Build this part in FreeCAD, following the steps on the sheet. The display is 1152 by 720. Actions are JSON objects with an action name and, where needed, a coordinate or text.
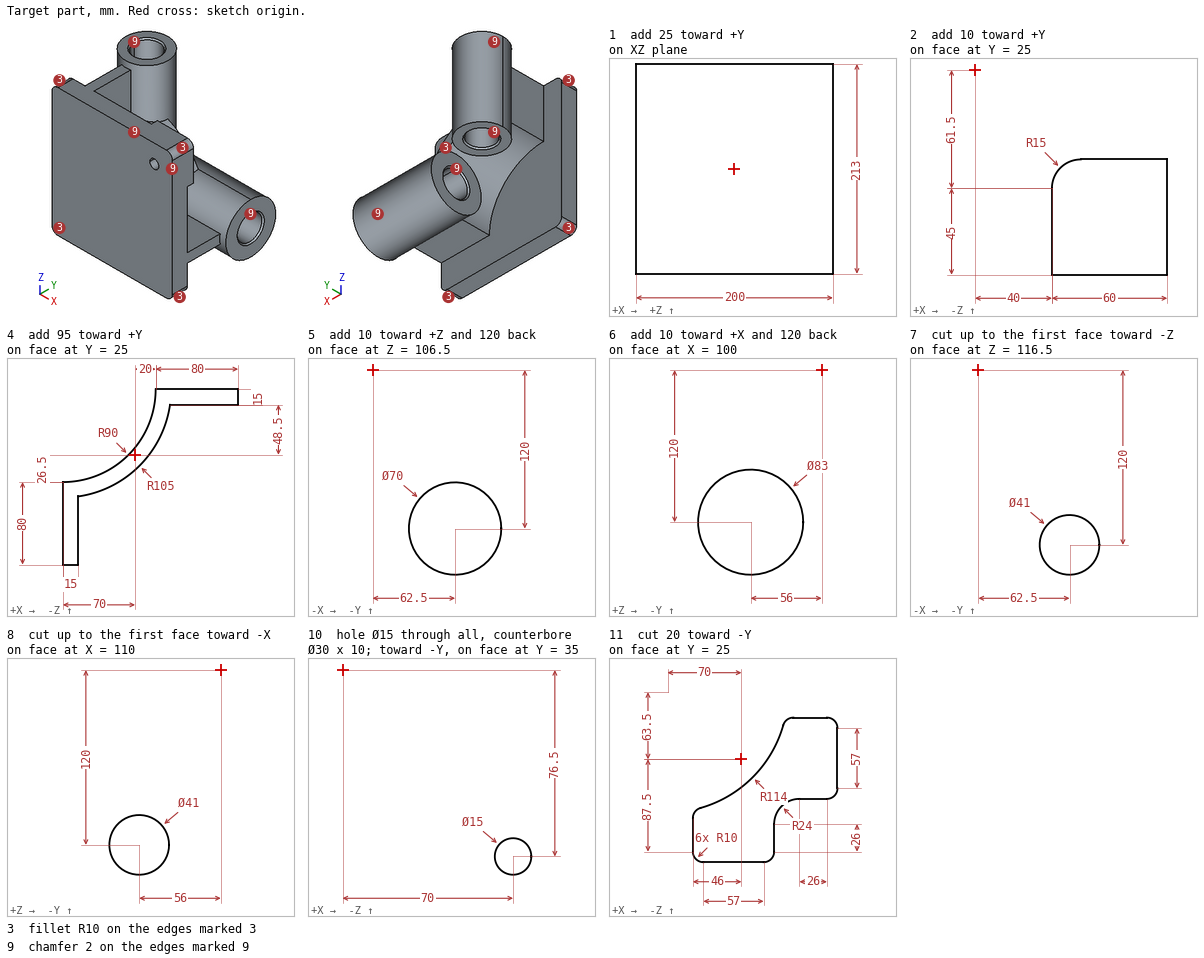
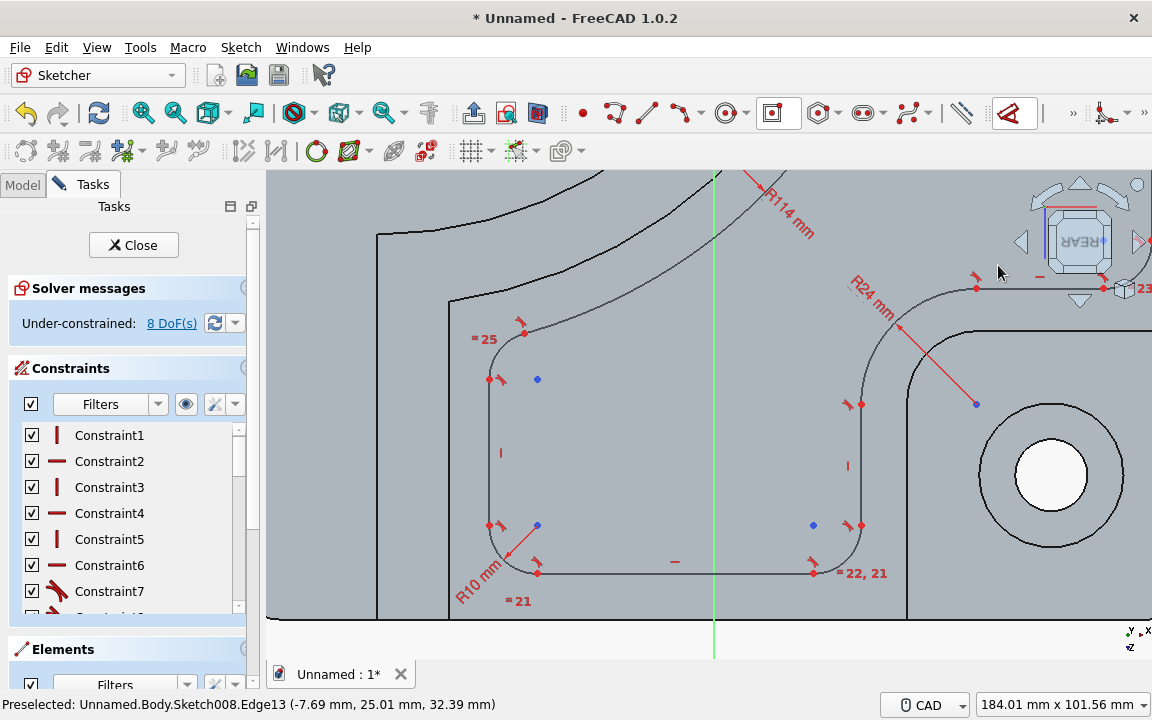
{"action": "left_click", "coordinate": [620, 574]}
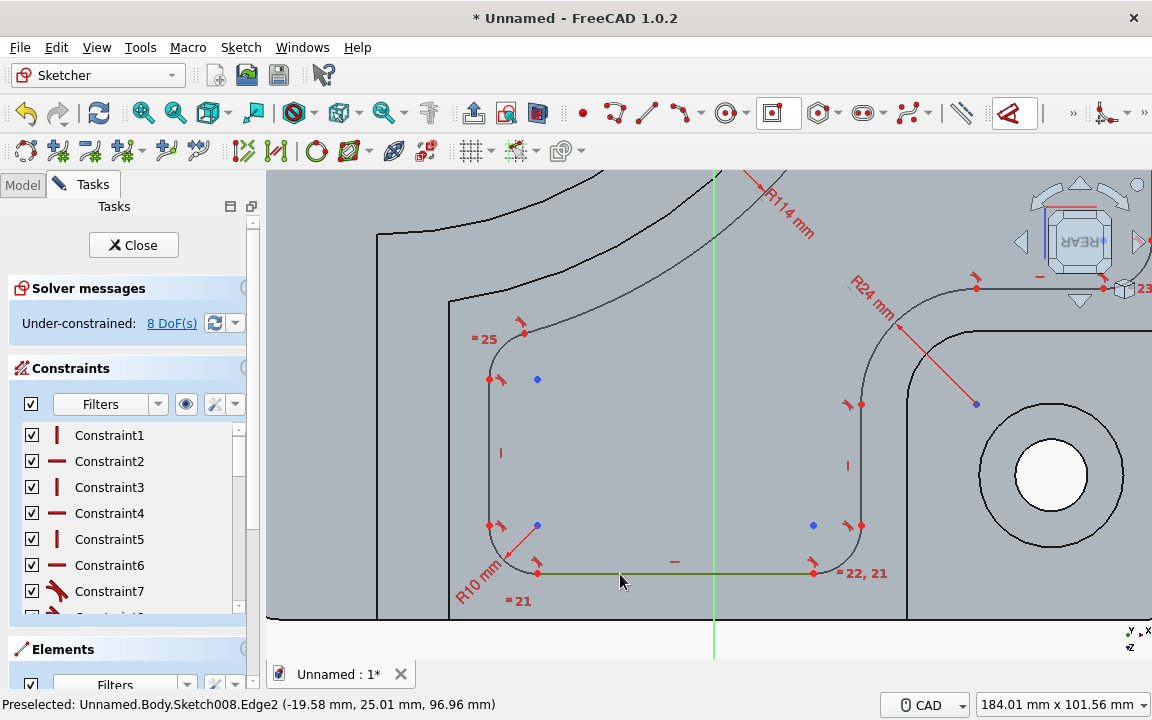
{"action": "key", "text": "l"}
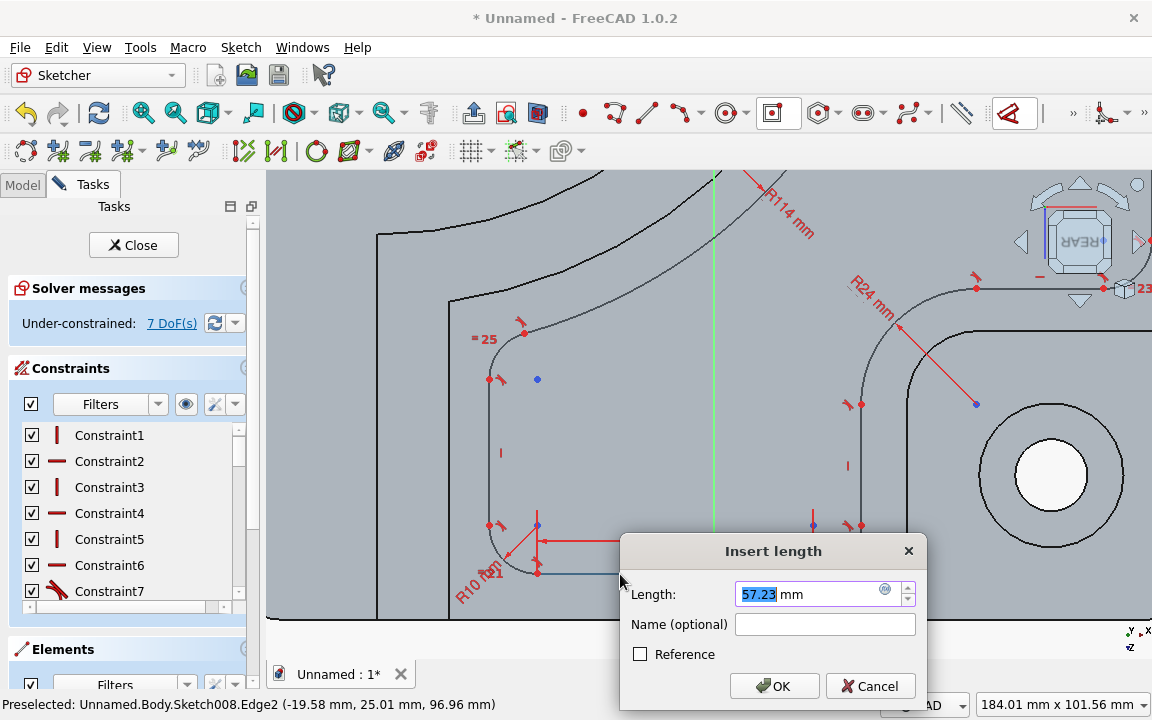
{"action": "type", "text": "57"}
{"action": "key", "text": "Return"}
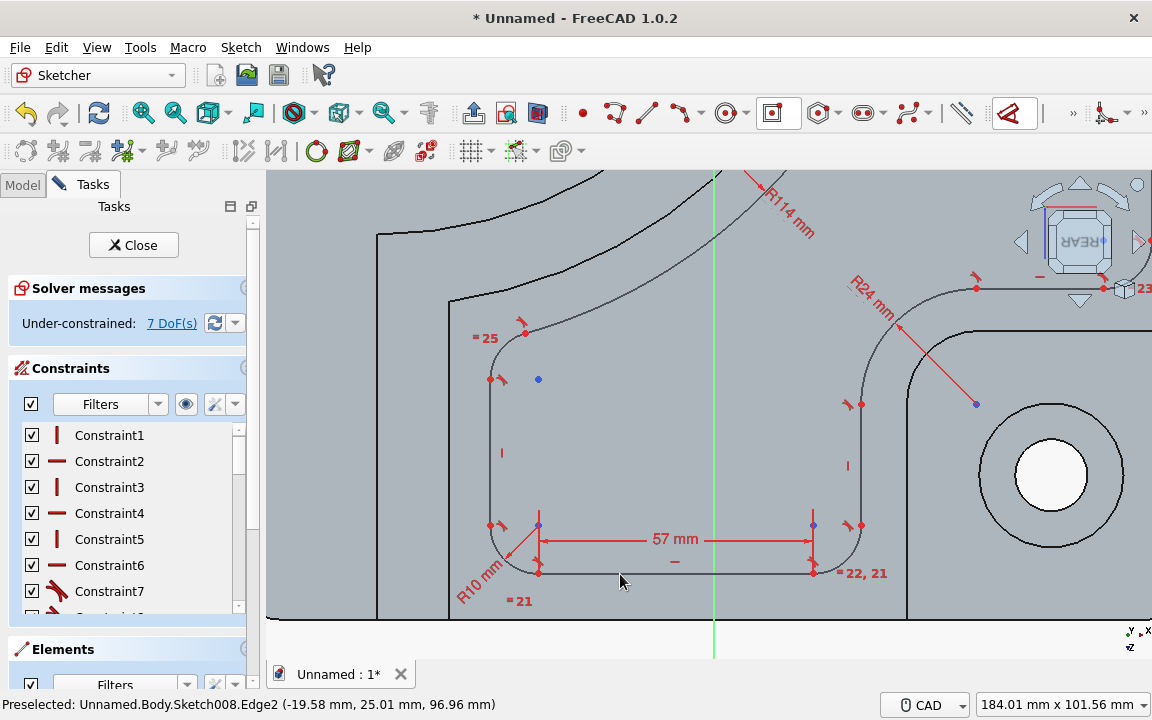
{"action": "left_click", "coordinate": [861, 489]}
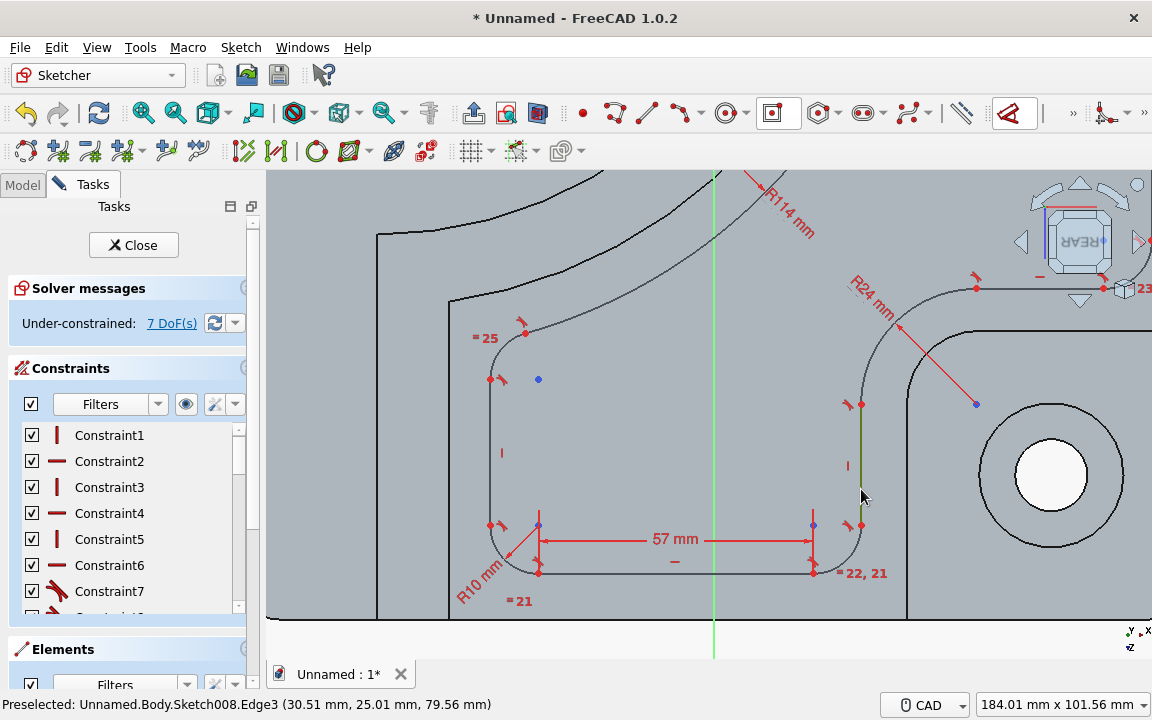
{"action": "left_click", "coordinate": [1032, 114]}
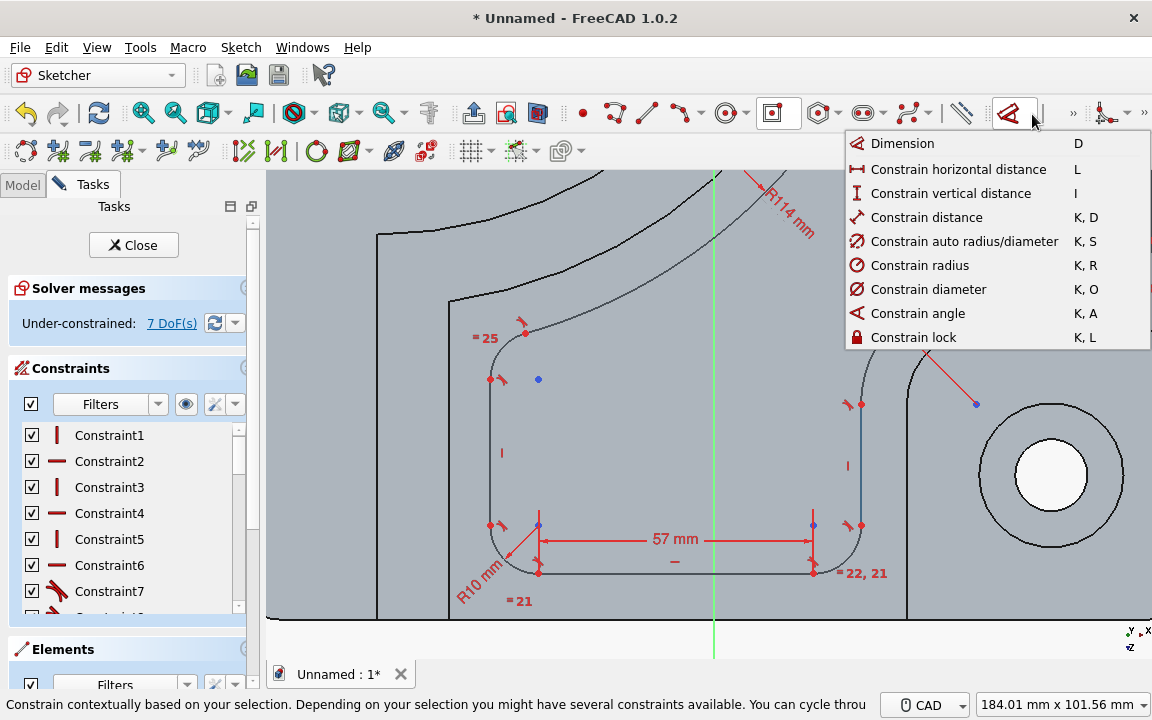
{"action": "left_click", "coordinate": [998, 193]}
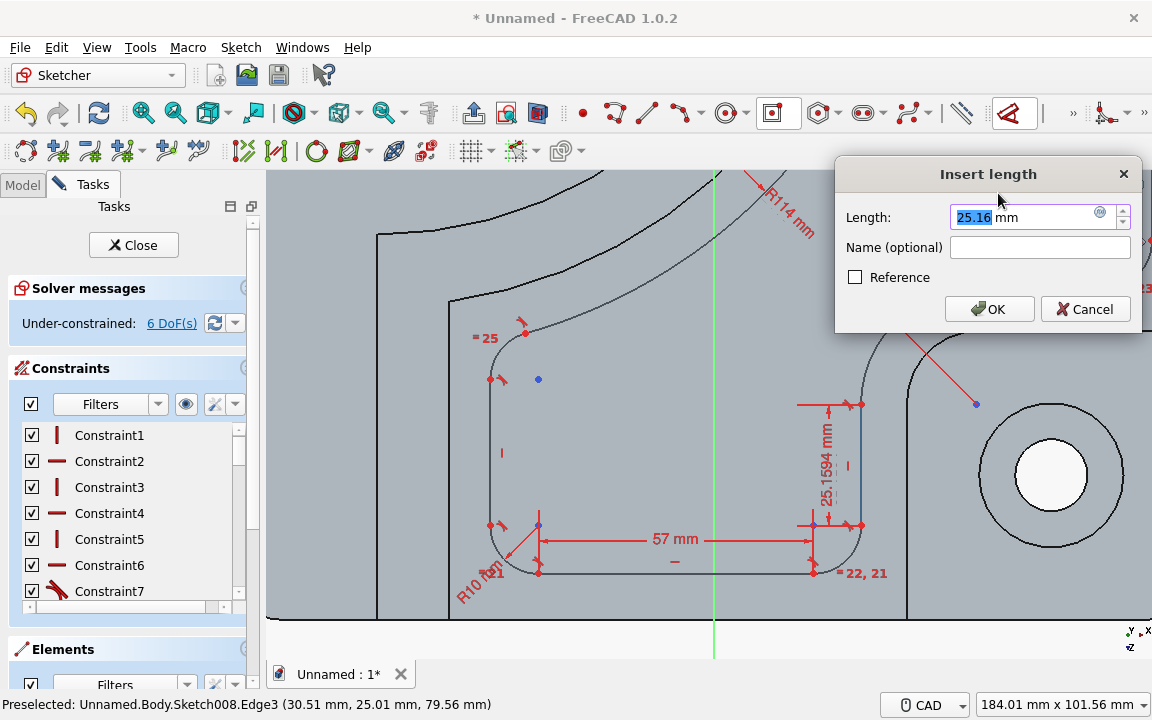
{"action": "type", "text": "26"}
{"action": "key", "text": "Return"}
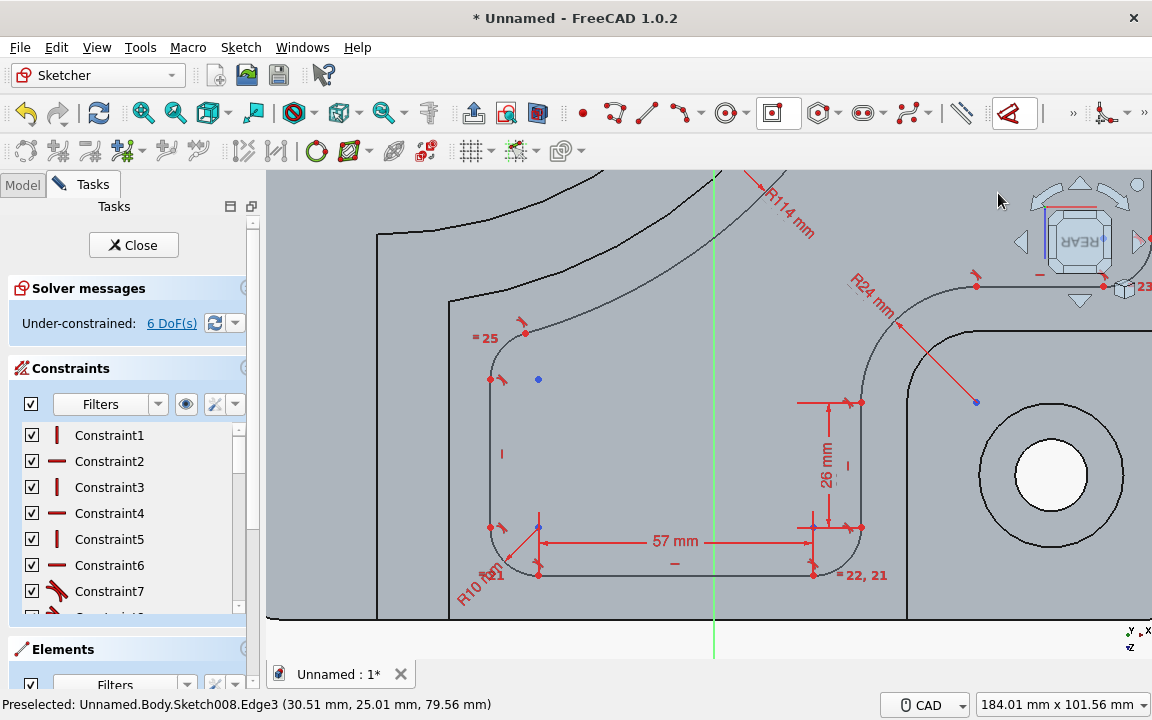
{"action": "scroll", "coordinate": [492, 552], "scroll_direction": "down", "scroll_amount": 4}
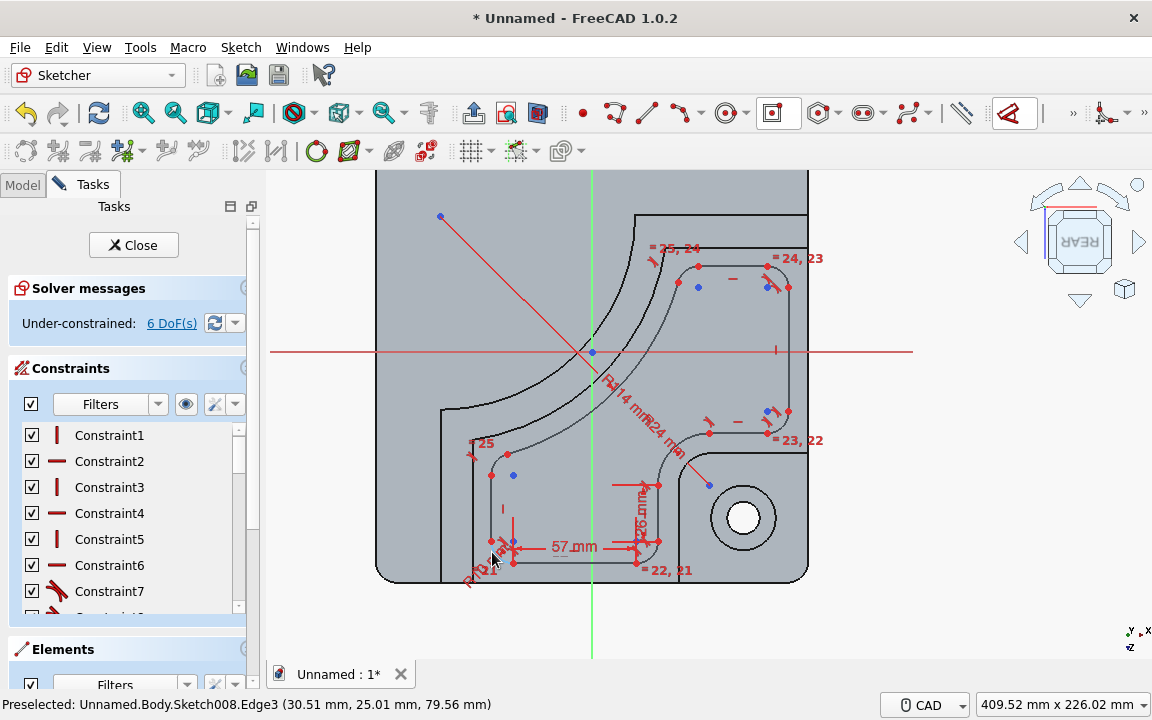
{"action": "left_click", "coordinate": [727, 433]}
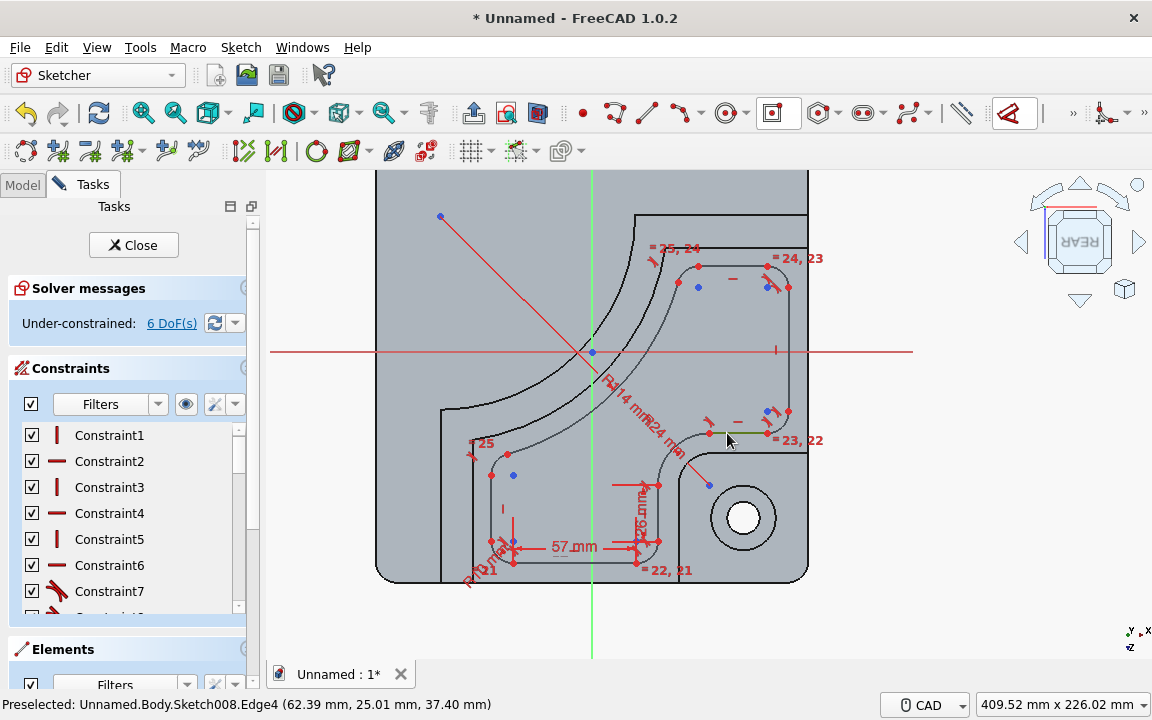
{"action": "key", "text": "l"}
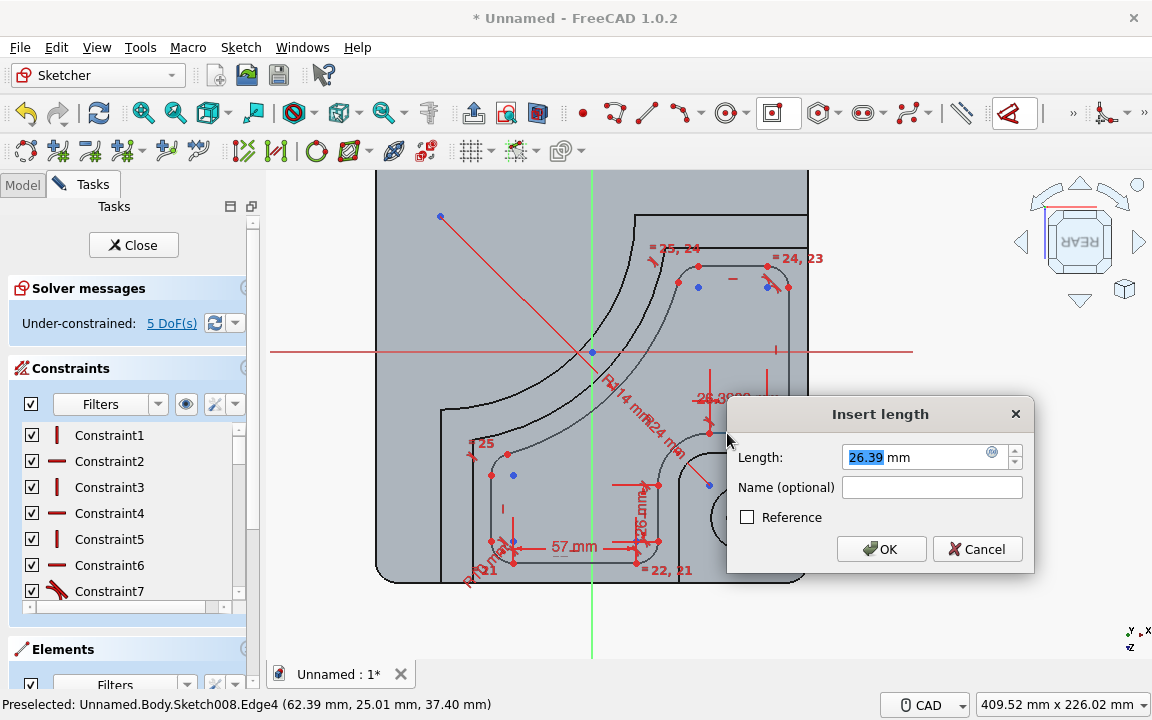
{"action": "type", "text": "26"}
{"action": "key", "text": "Return"}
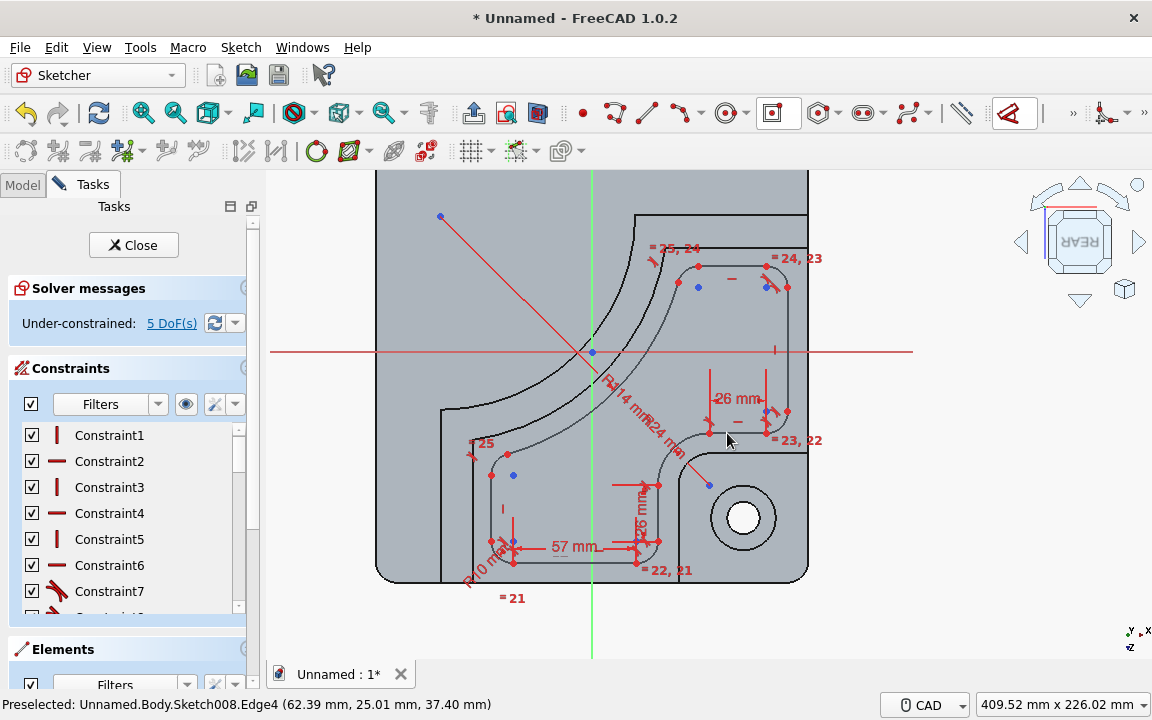
{"action": "left_click", "coordinate": [788, 375]}